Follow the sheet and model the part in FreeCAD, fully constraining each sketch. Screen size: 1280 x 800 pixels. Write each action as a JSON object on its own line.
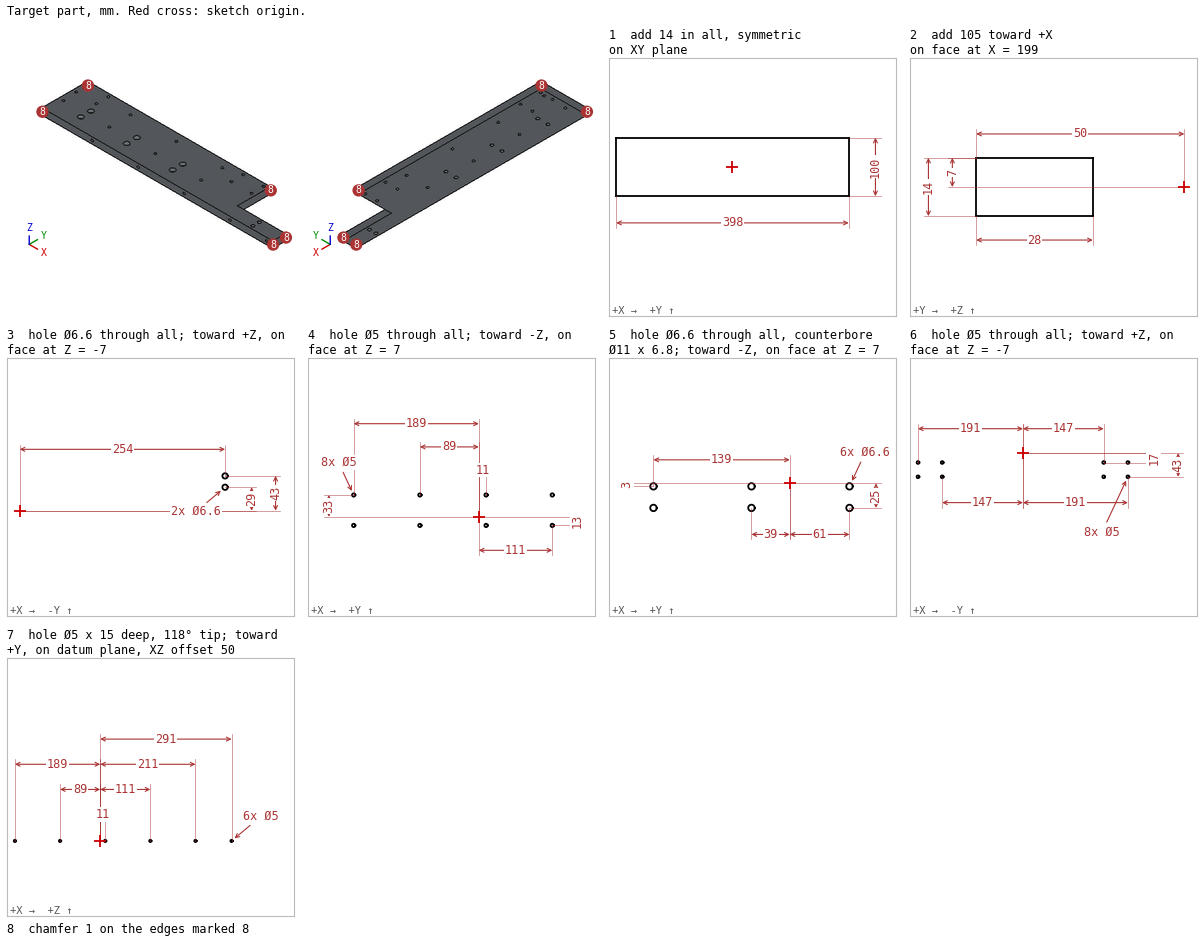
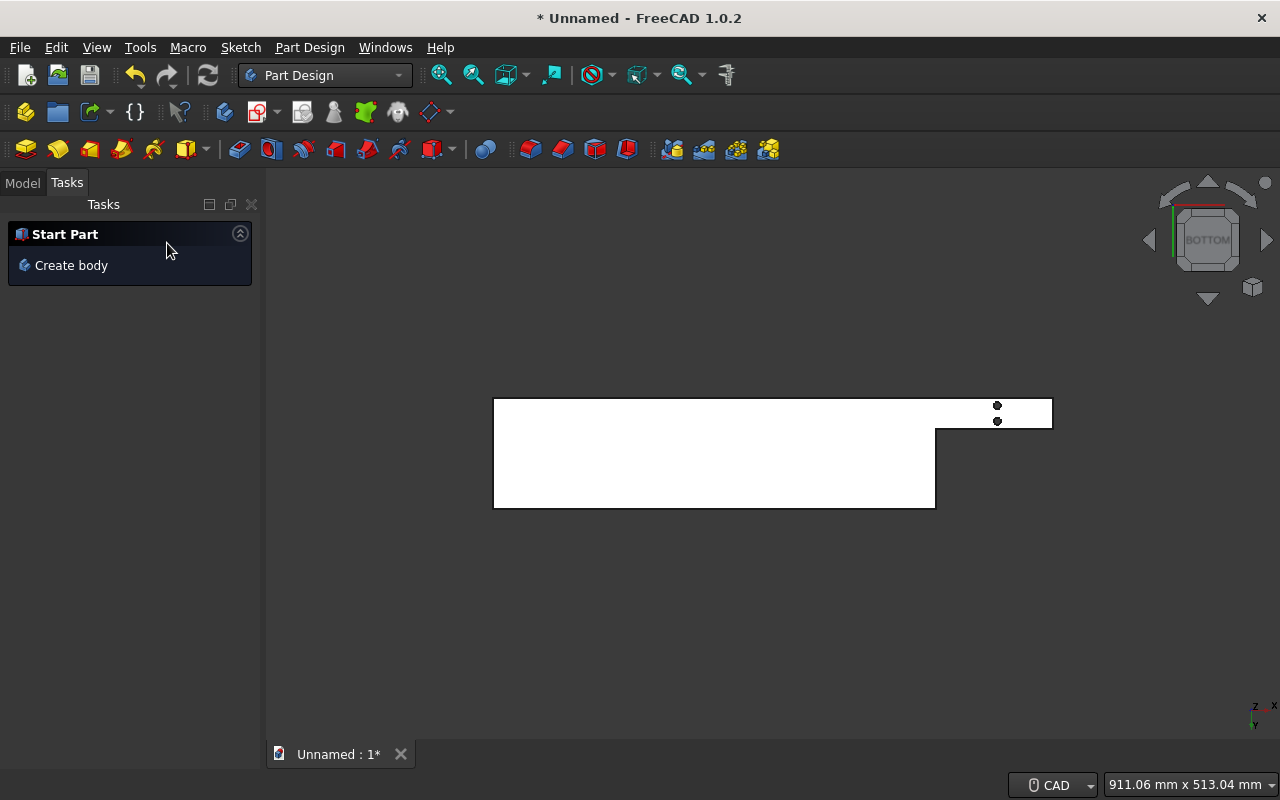
{"action": "key", "text": "0"}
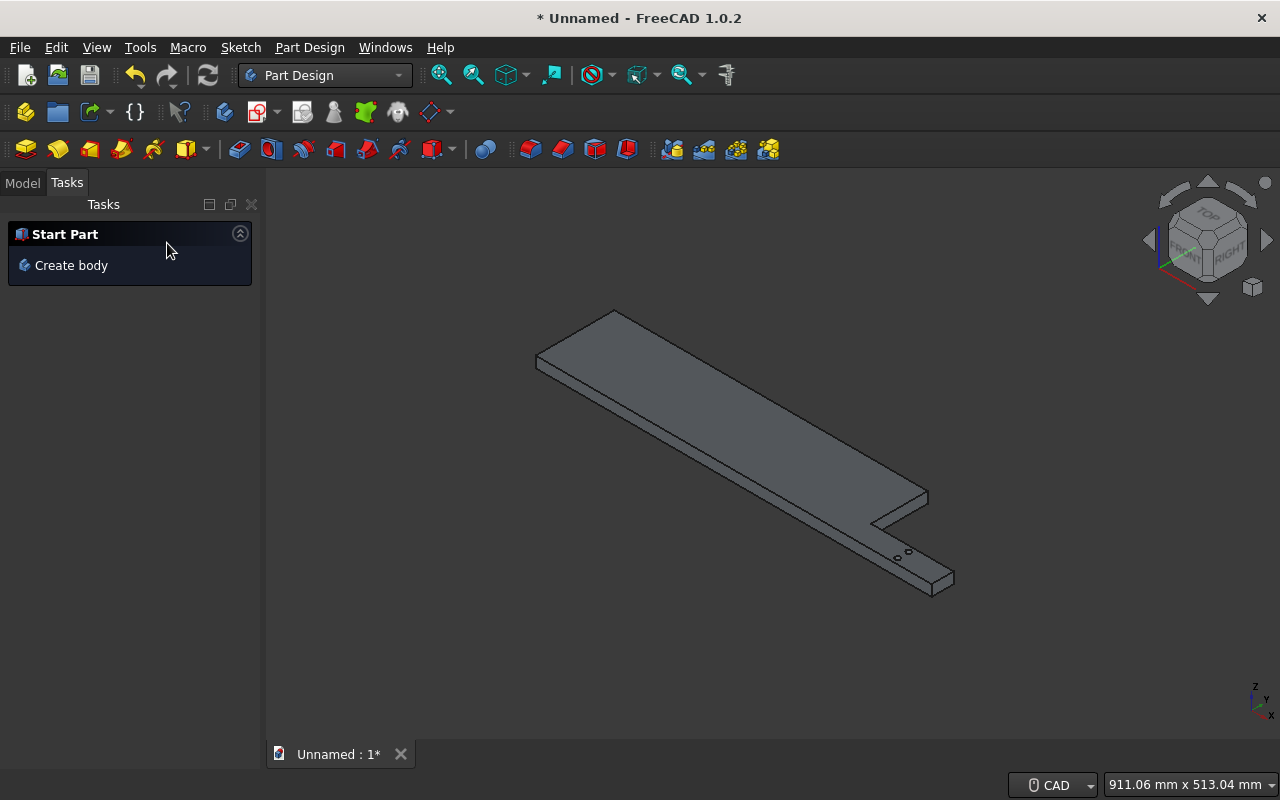
{"action": "left_click", "coordinate": [830, 479]}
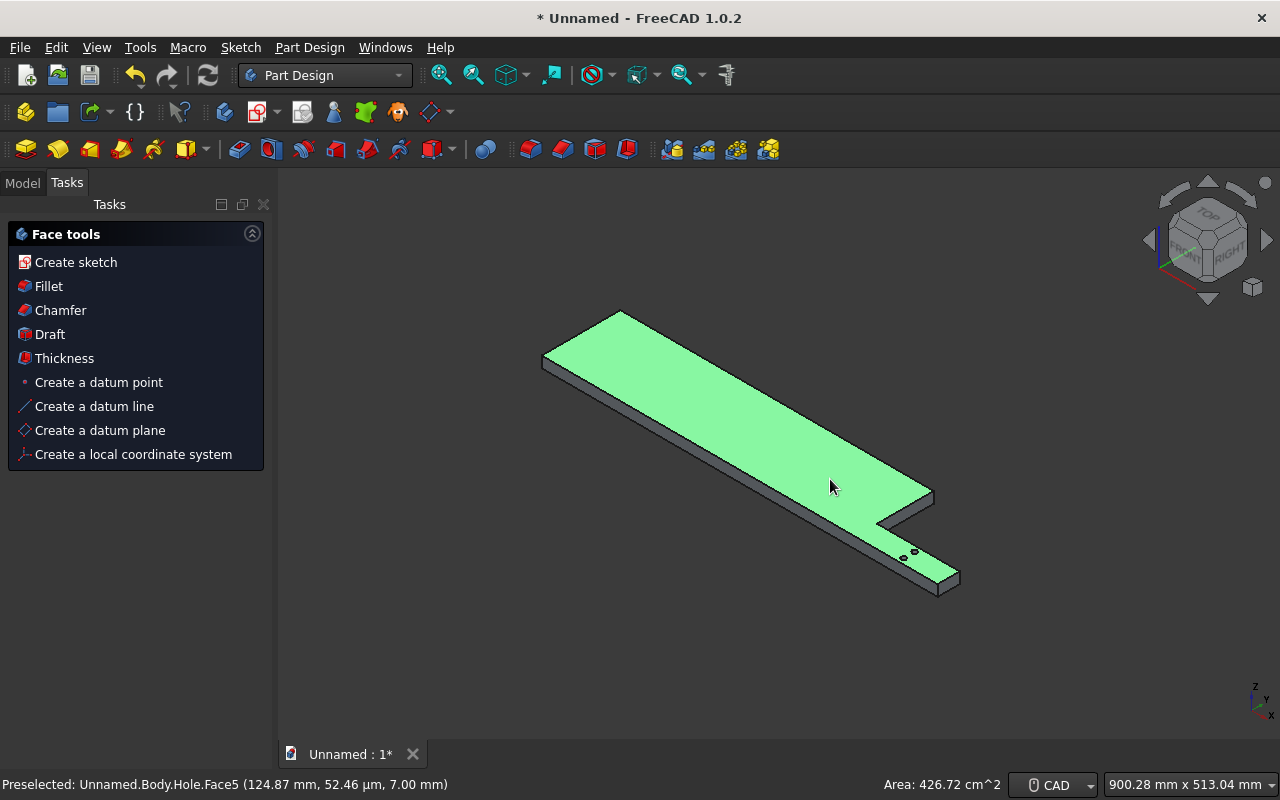
{"action": "left_click", "coordinate": [258, 112]}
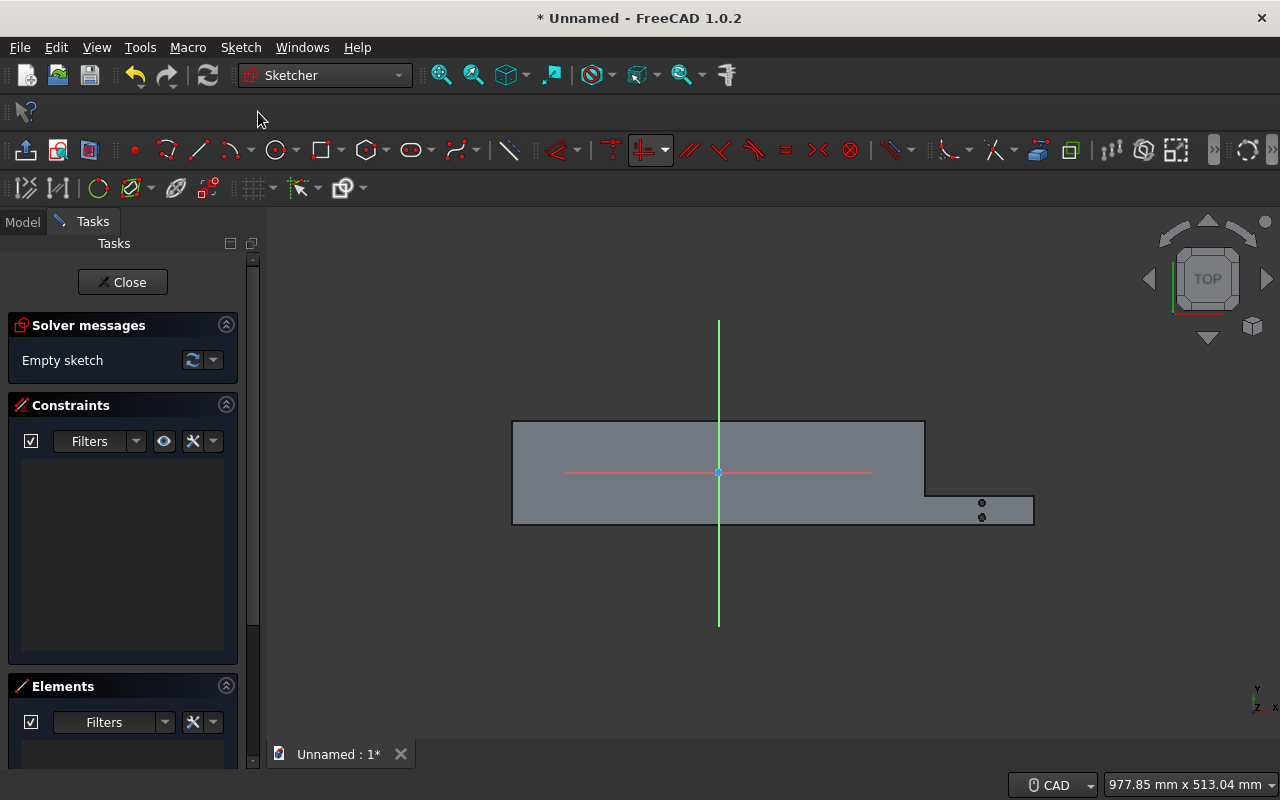
{"action": "scroll", "coordinate": [646, 450], "scroll_direction": "up", "scroll_amount": 3}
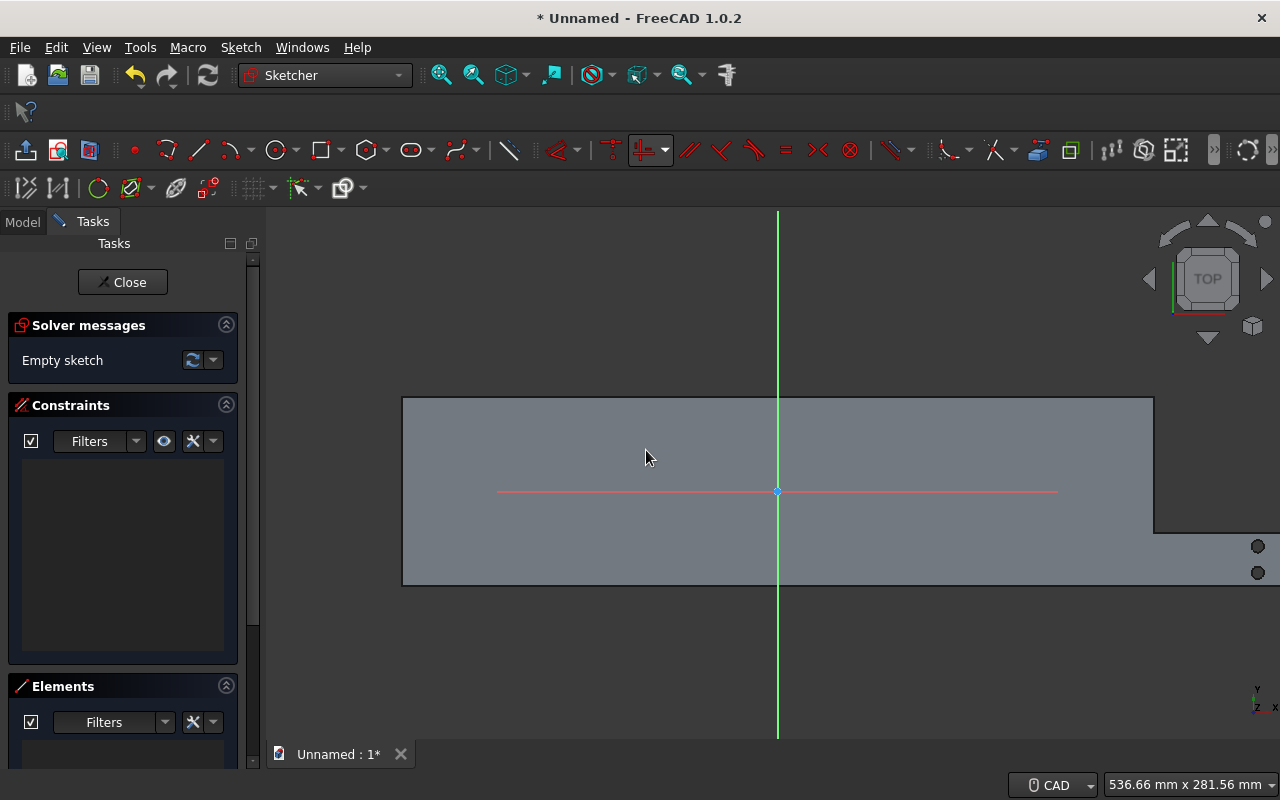
{"action": "left_click", "coordinate": [276, 150]}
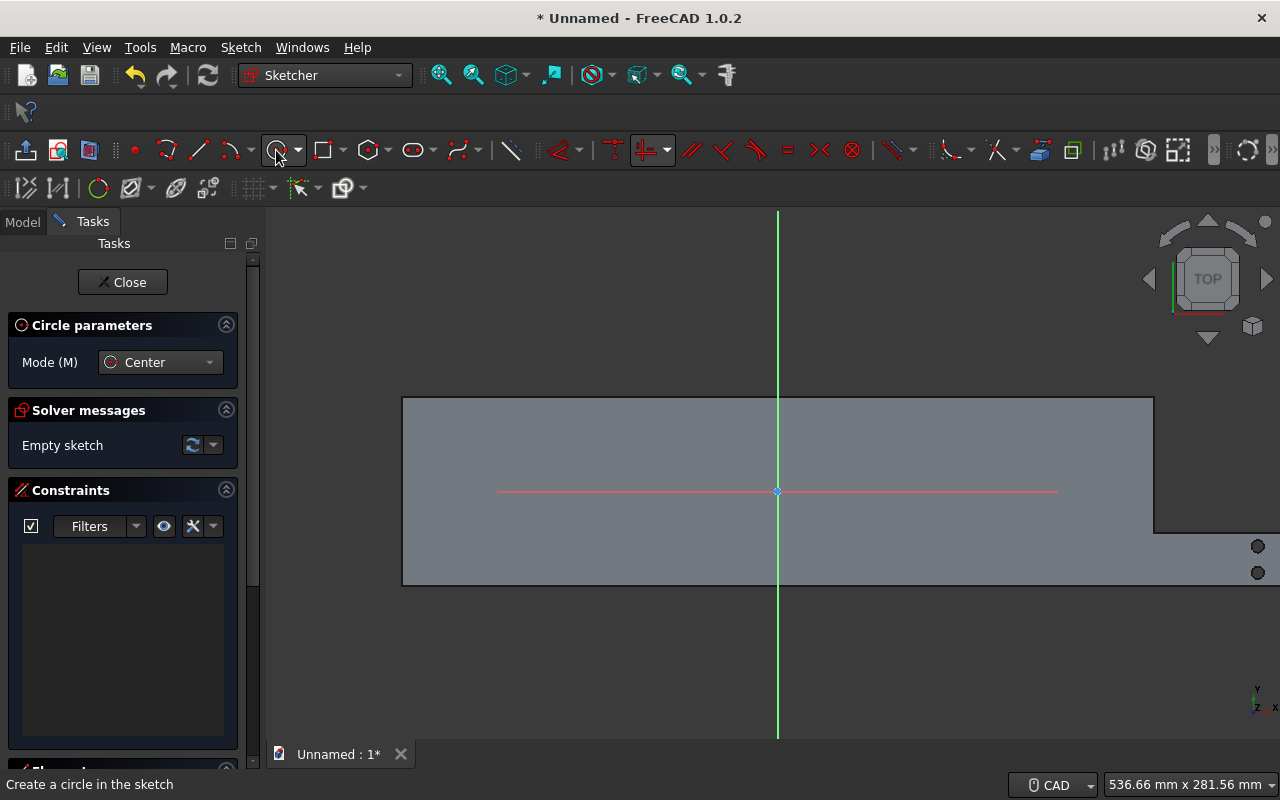
{"action": "scroll", "coordinate": [988, 516], "scroll_direction": "up", "scroll_amount": 8}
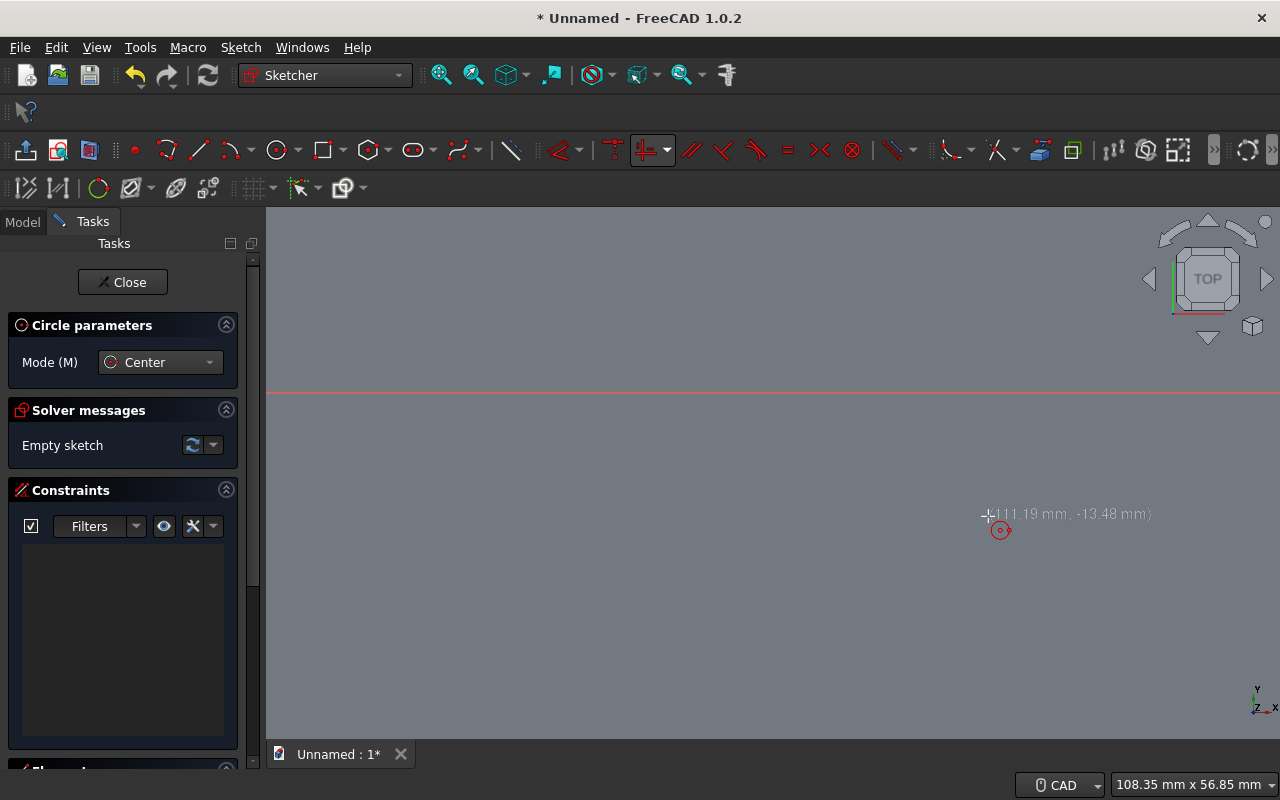
{"action": "scroll", "coordinate": [989, 517], "scroll_direction": "down", "scroll_amount": 8}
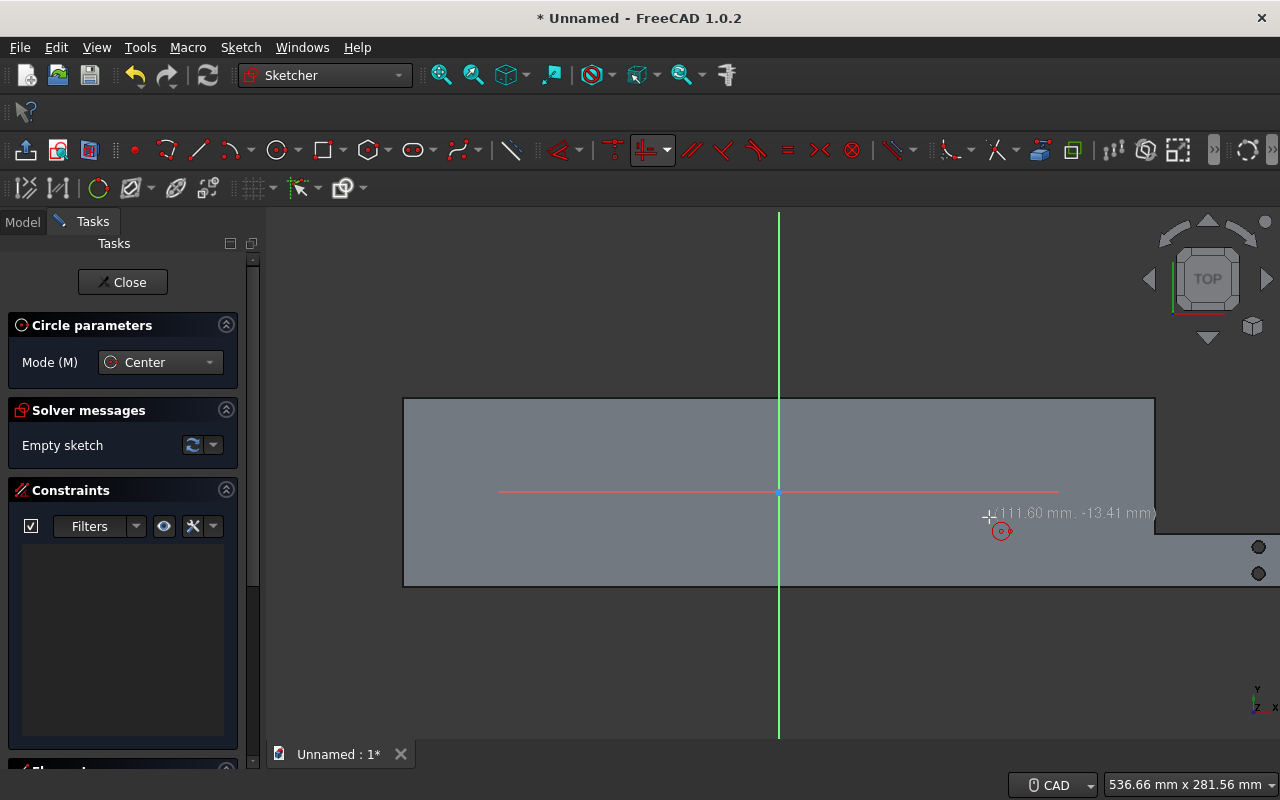
{"action": "left_click", "coordinate": [988, 517]}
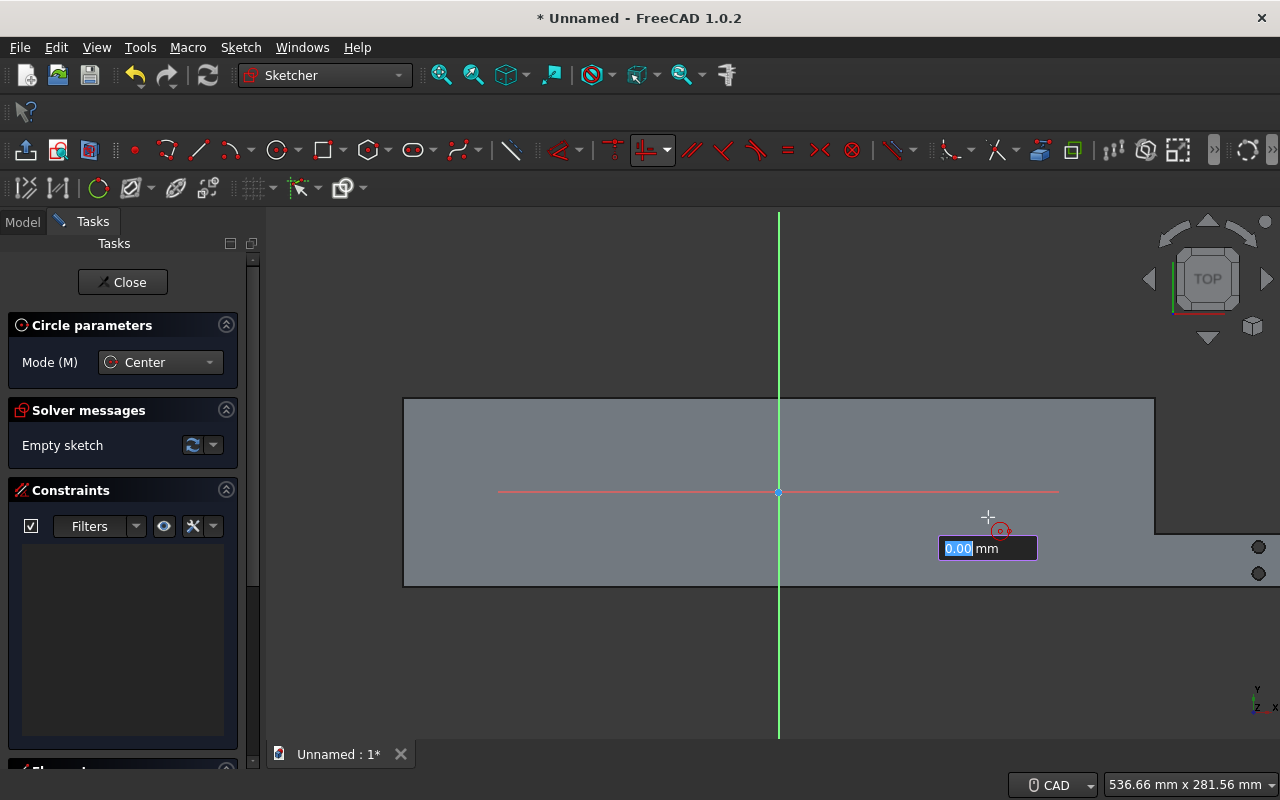
{"action": "scroll", "coordinate": [992, 514], "scroll_direction": "up", "scroll_amount": 7}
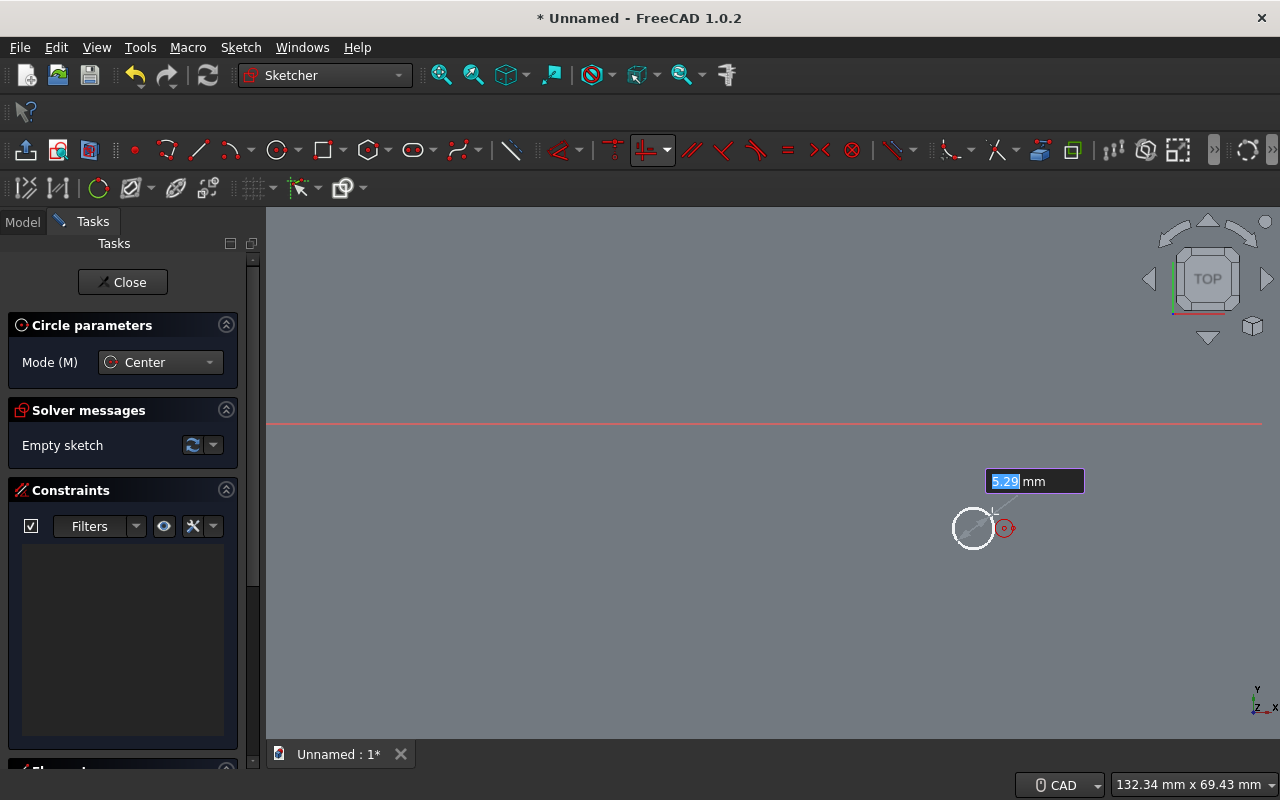
{"action": "left_click", "coordinate": [989, 510]}